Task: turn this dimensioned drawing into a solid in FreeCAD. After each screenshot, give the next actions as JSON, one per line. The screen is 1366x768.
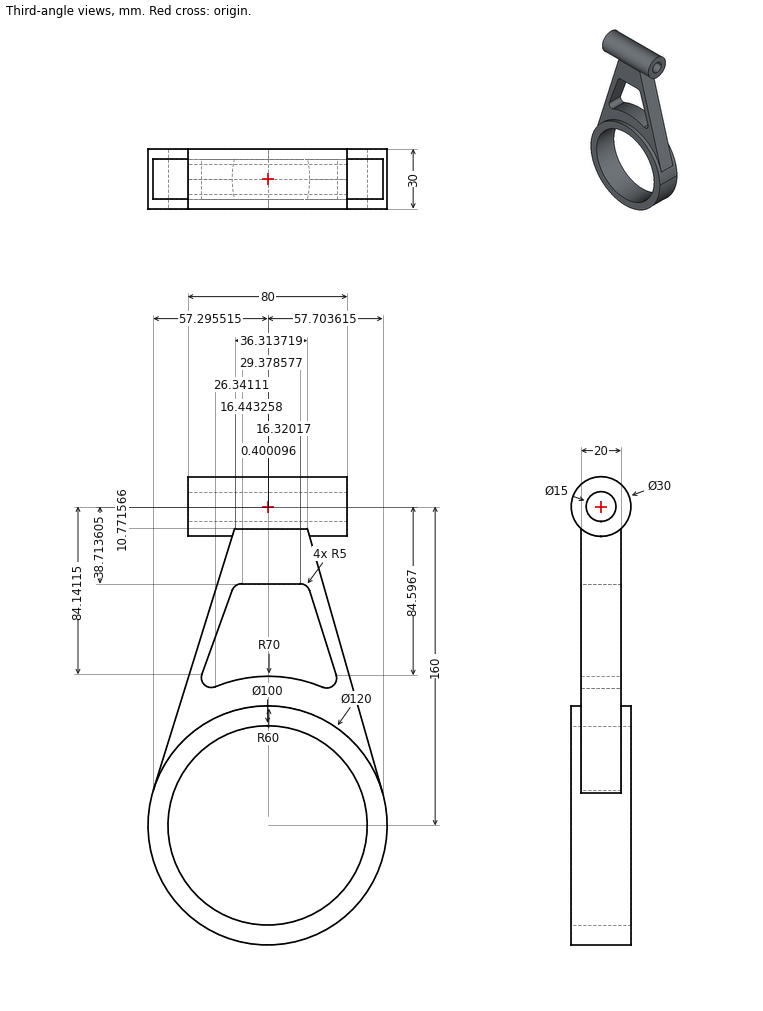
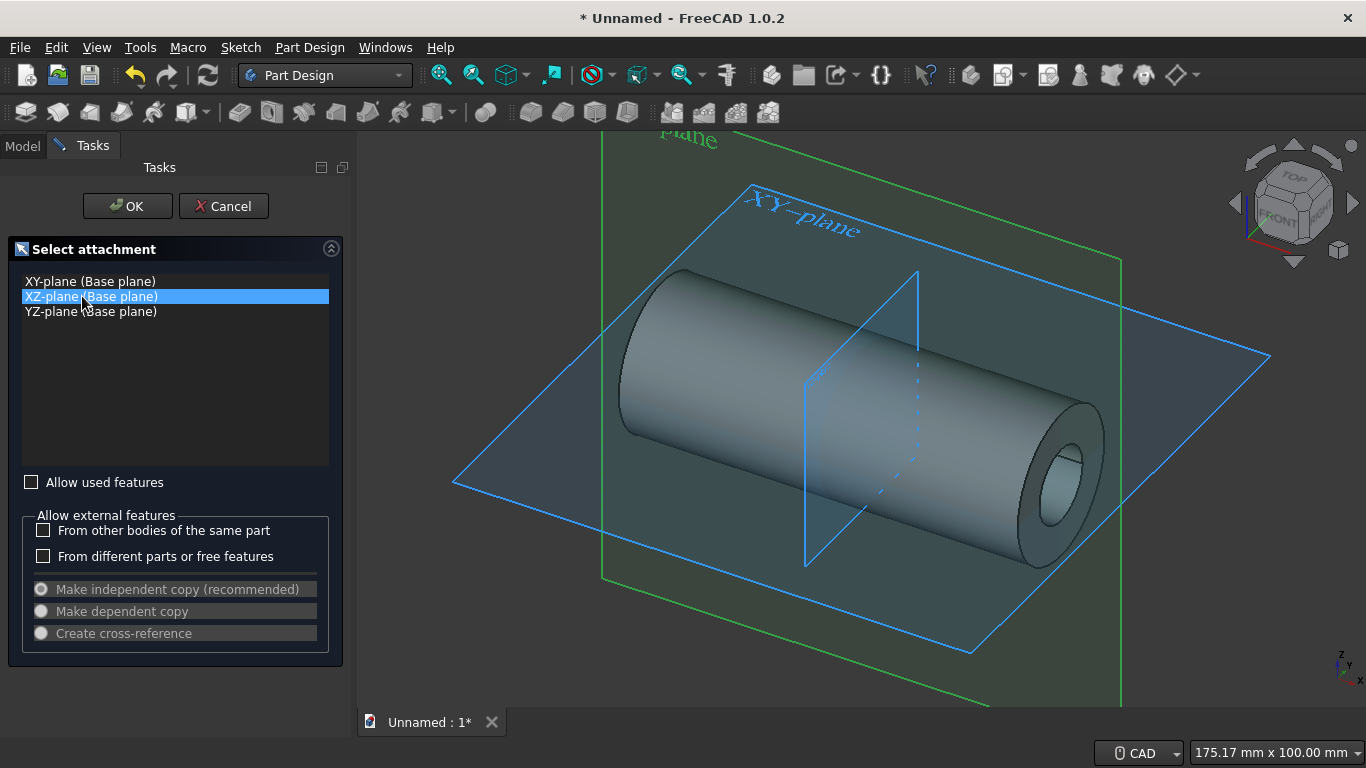
{"action": "left_click", "coordinate": [128, 206]}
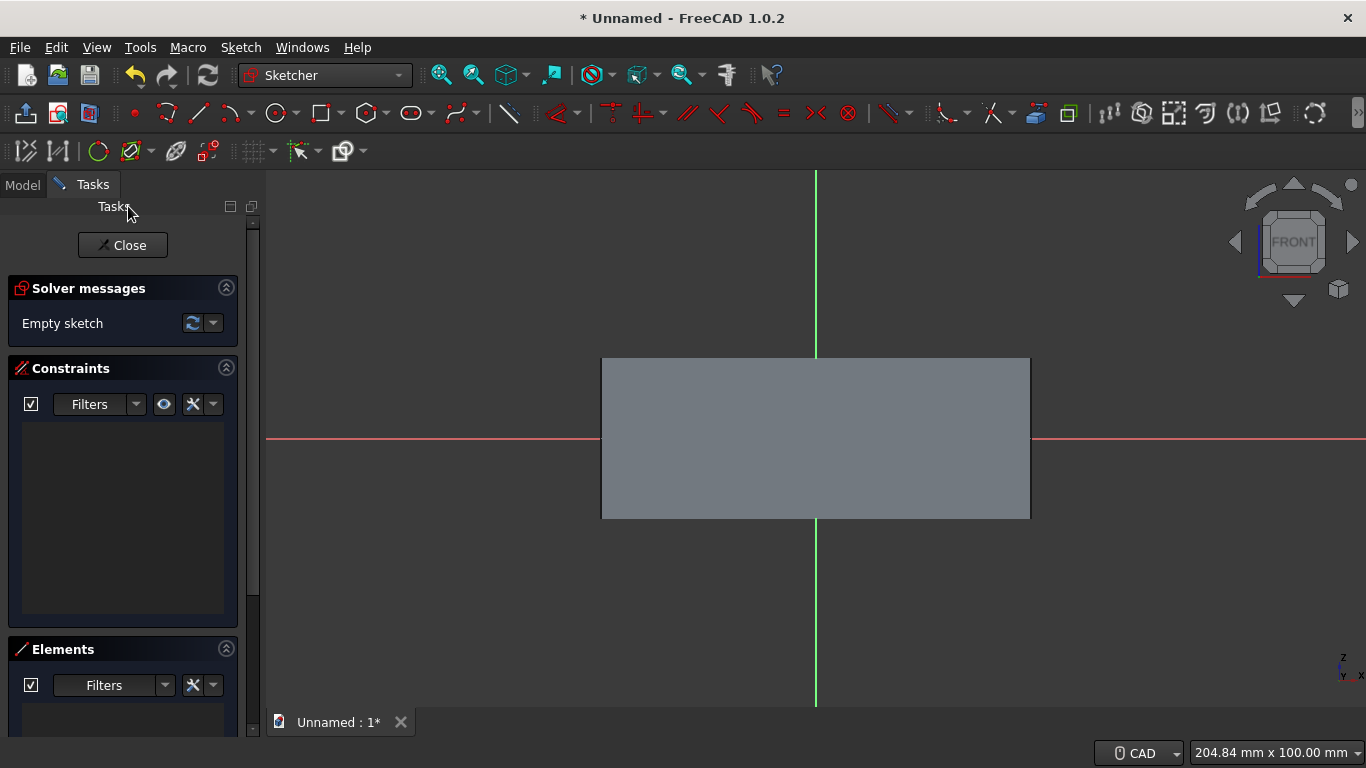
{"action": "key", "text": "q s"}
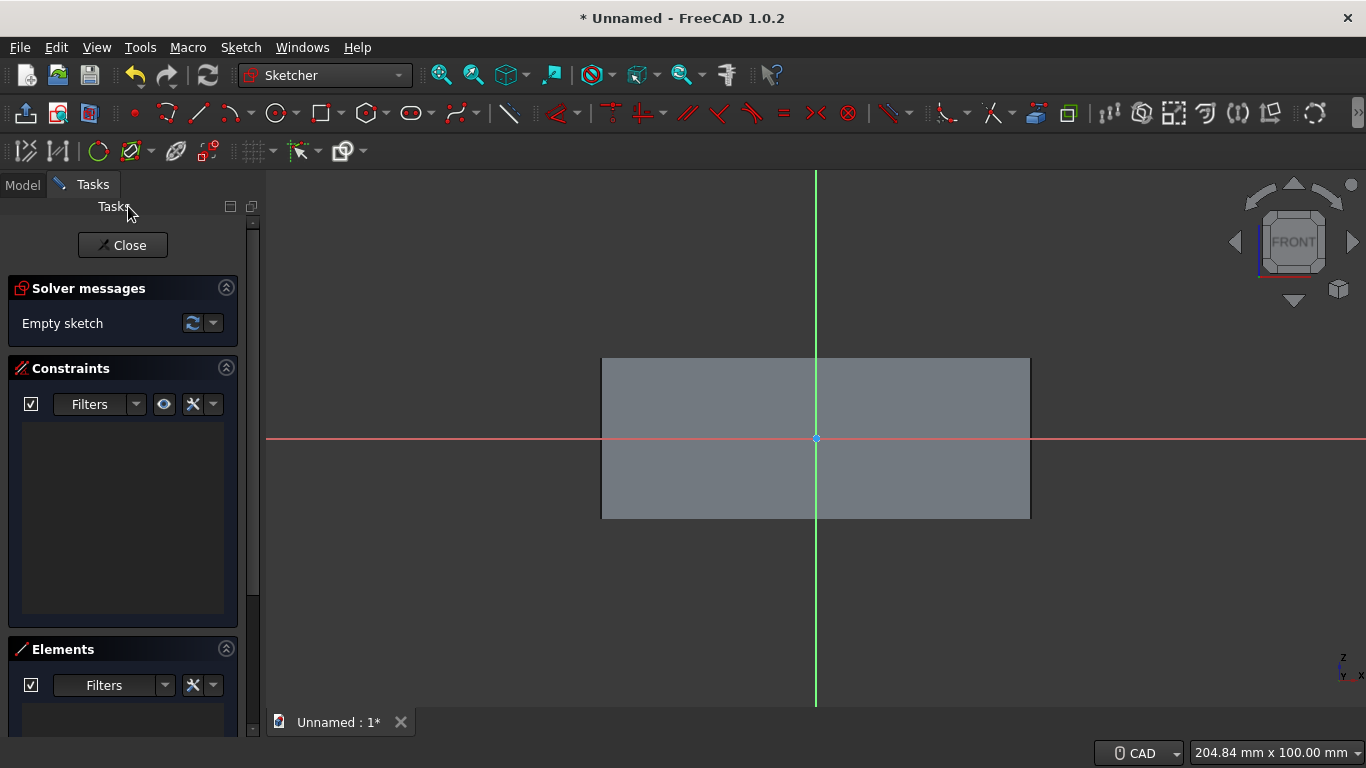
{"action": "scroll", "coordinate": [691, 198], "scroll_direction": "down", "scroll_amount": 4}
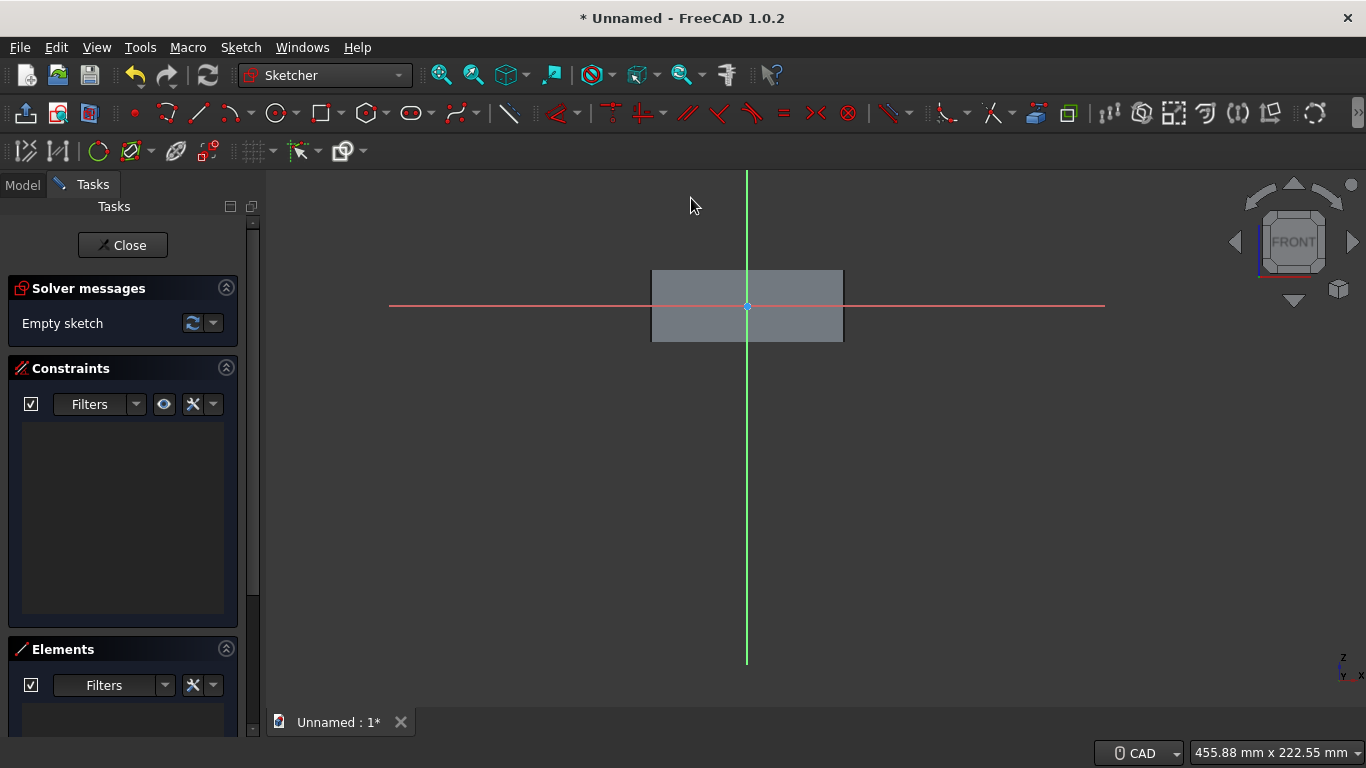
{"action": "key", "text": "g m"}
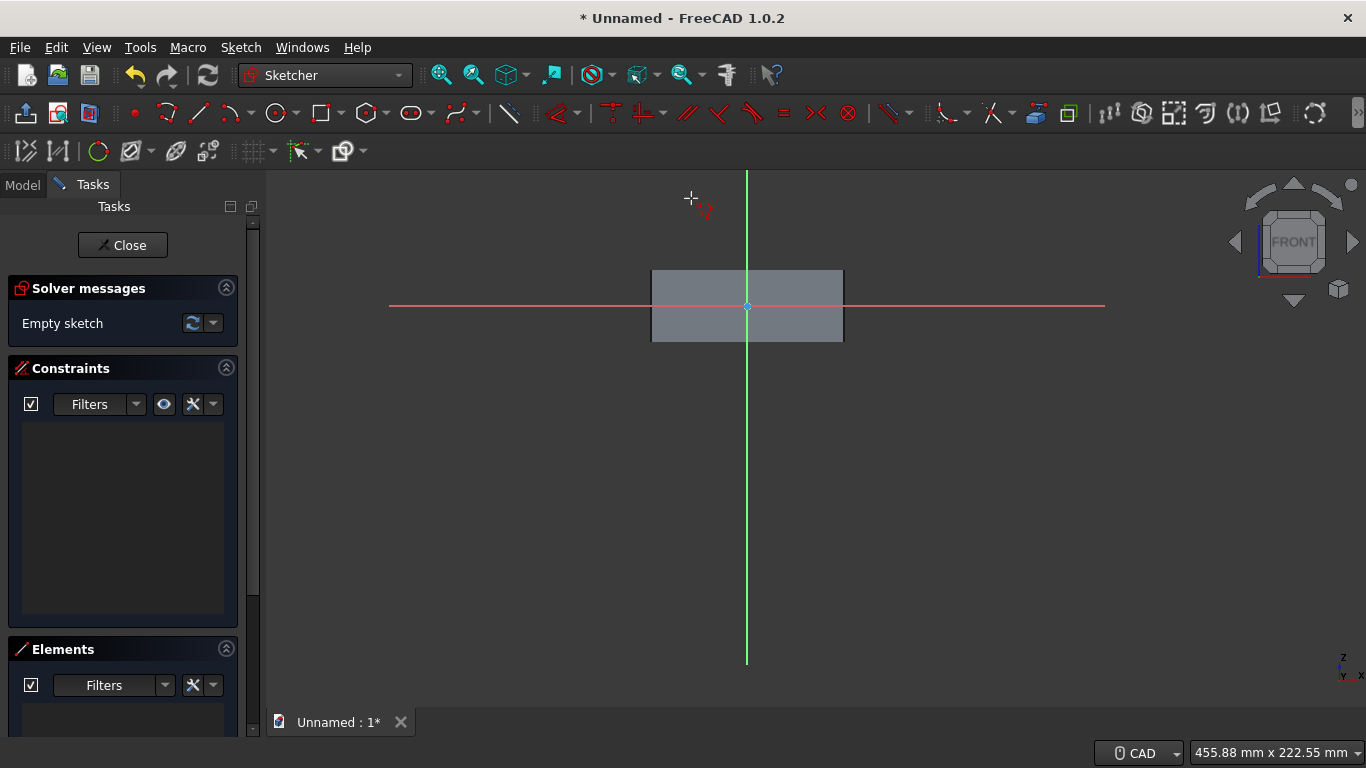
{"action": "left_click", "coordinate": [609, 649]}
{"action": "left_click", "coordinate": [708, 332]}
{"action": "left_click", "coordinate": [795, 332]}
{"action": "left_click", "coordinate": [887, 652]}
{"action": "right_click", "coordinate": [887, 652]}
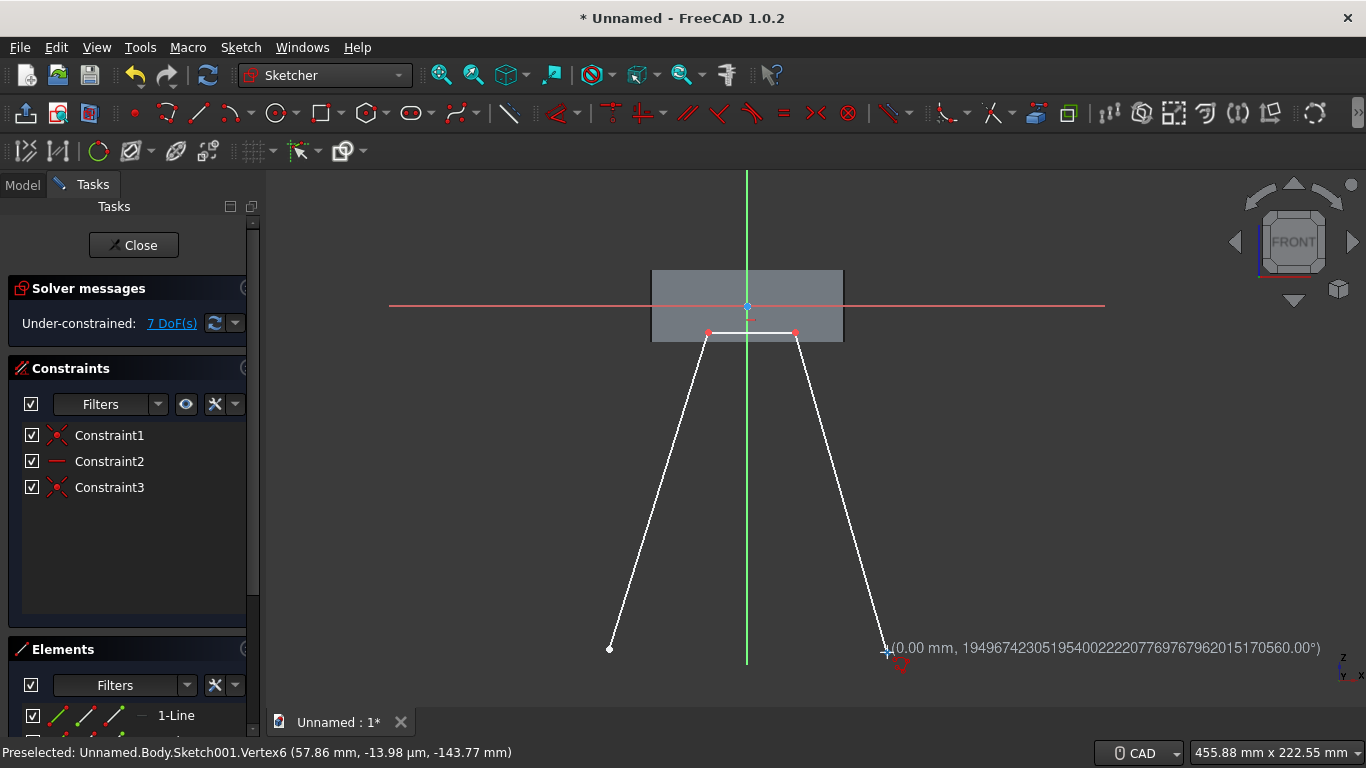
{"action": "key", "text": "g 3 a"}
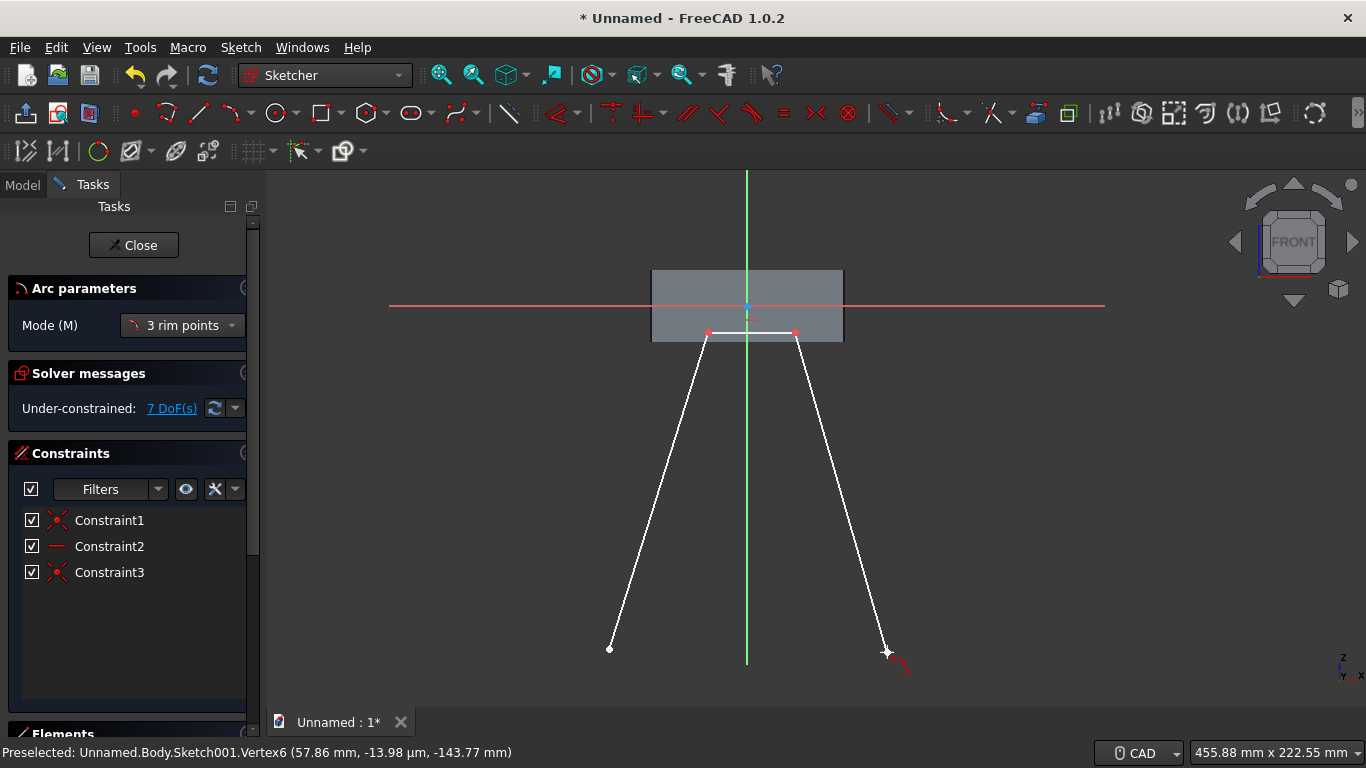
{"action": "left_click", "coordinate": [887, 653]}
{"action": "left_click", "coordinate": [609, 650]}
{"action": "left_click", "coordinate": [786, 553]}
{"action": "key", "text": "Escape"}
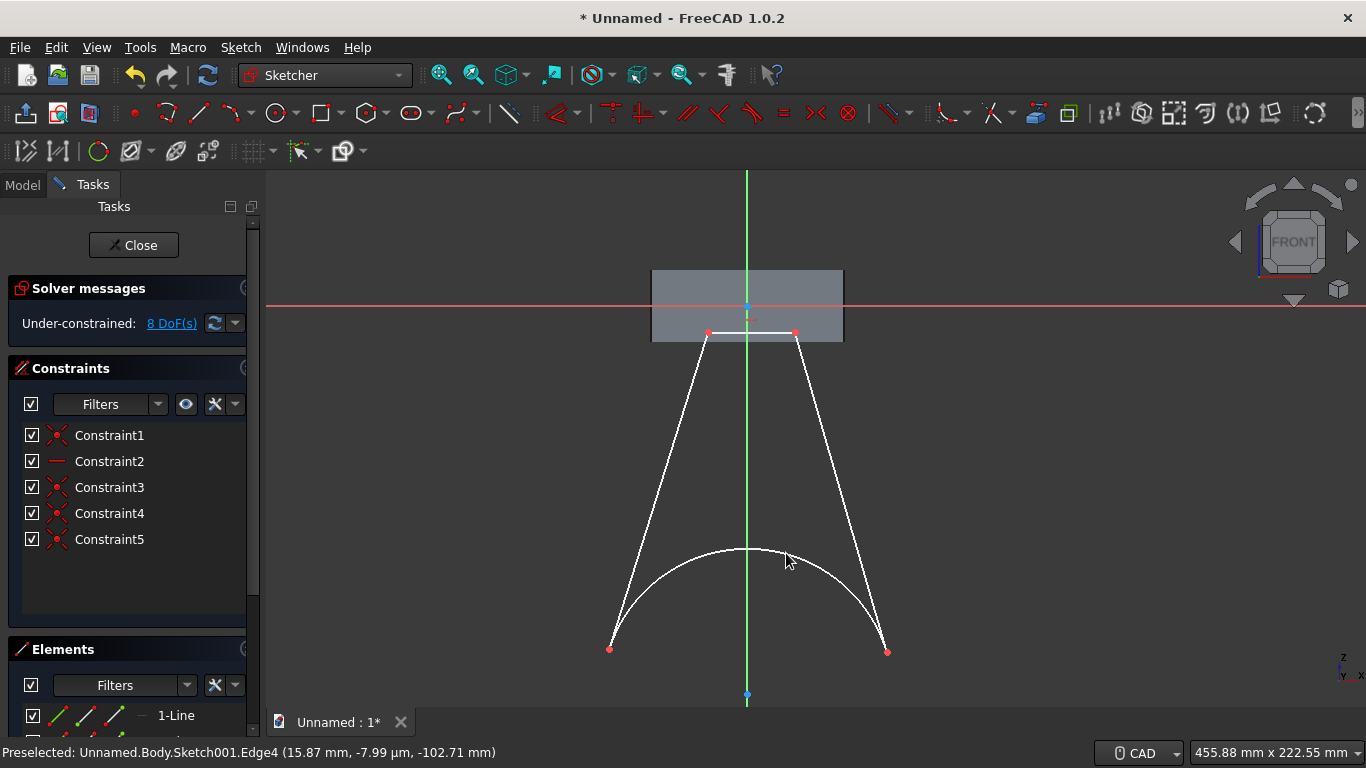
{"action": "scroll", "coordinate": [746, 198], "scroll_direction": "down", "scroll_amount": 1}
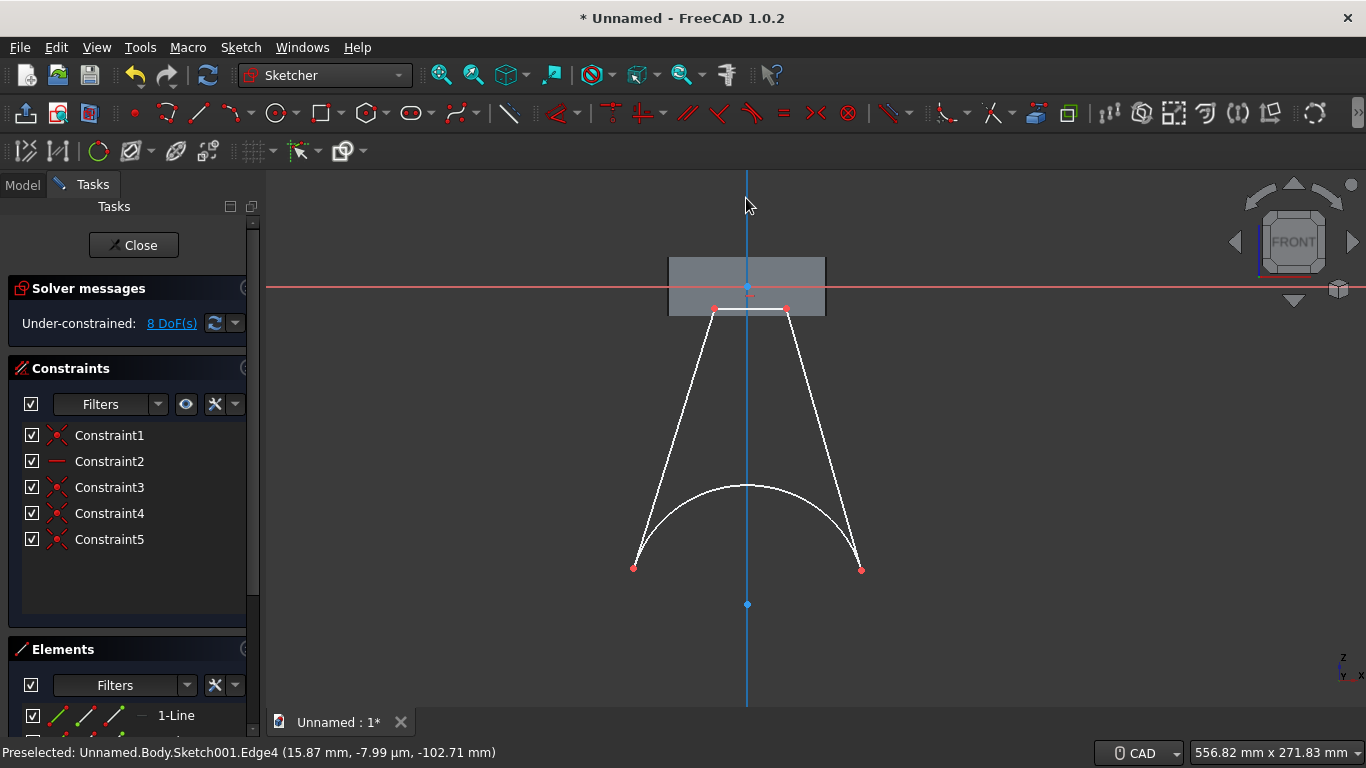
{"action": "left_click", "coordinate": [747, 604]}